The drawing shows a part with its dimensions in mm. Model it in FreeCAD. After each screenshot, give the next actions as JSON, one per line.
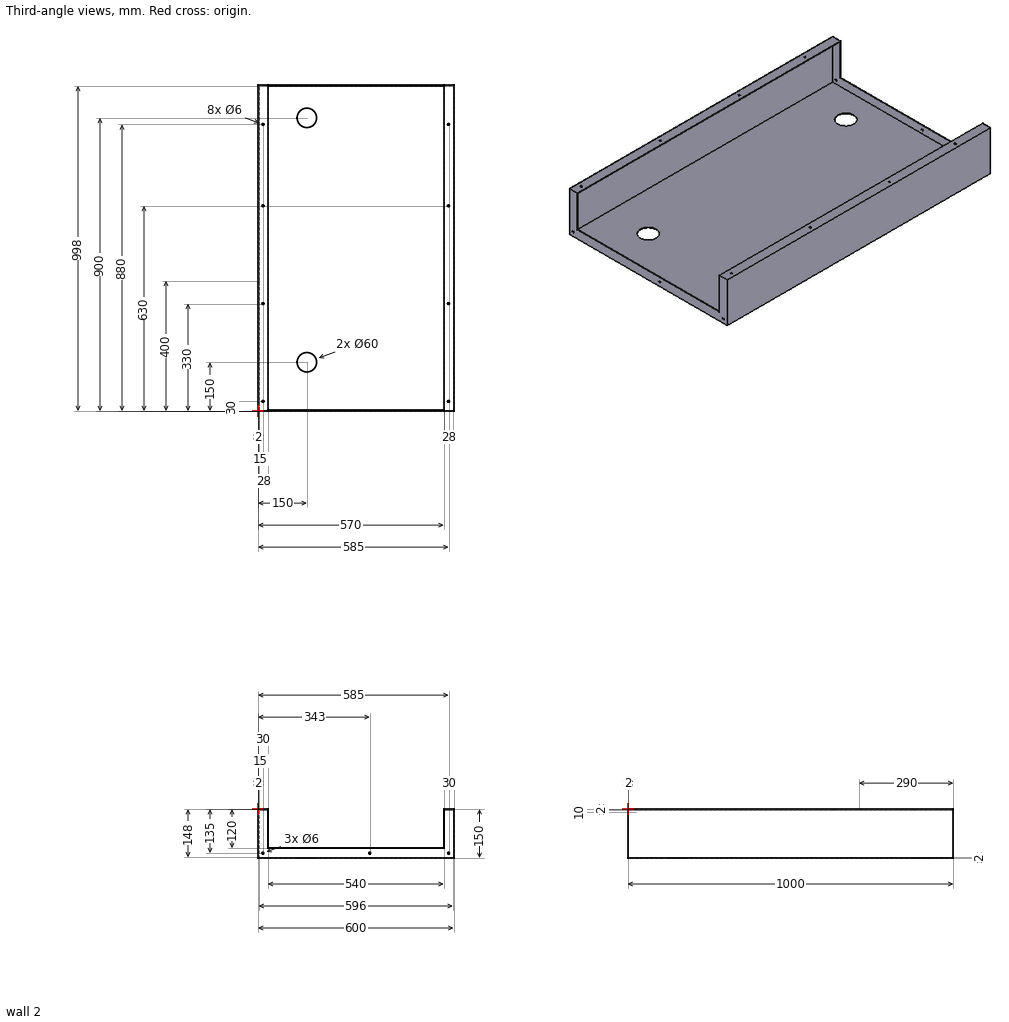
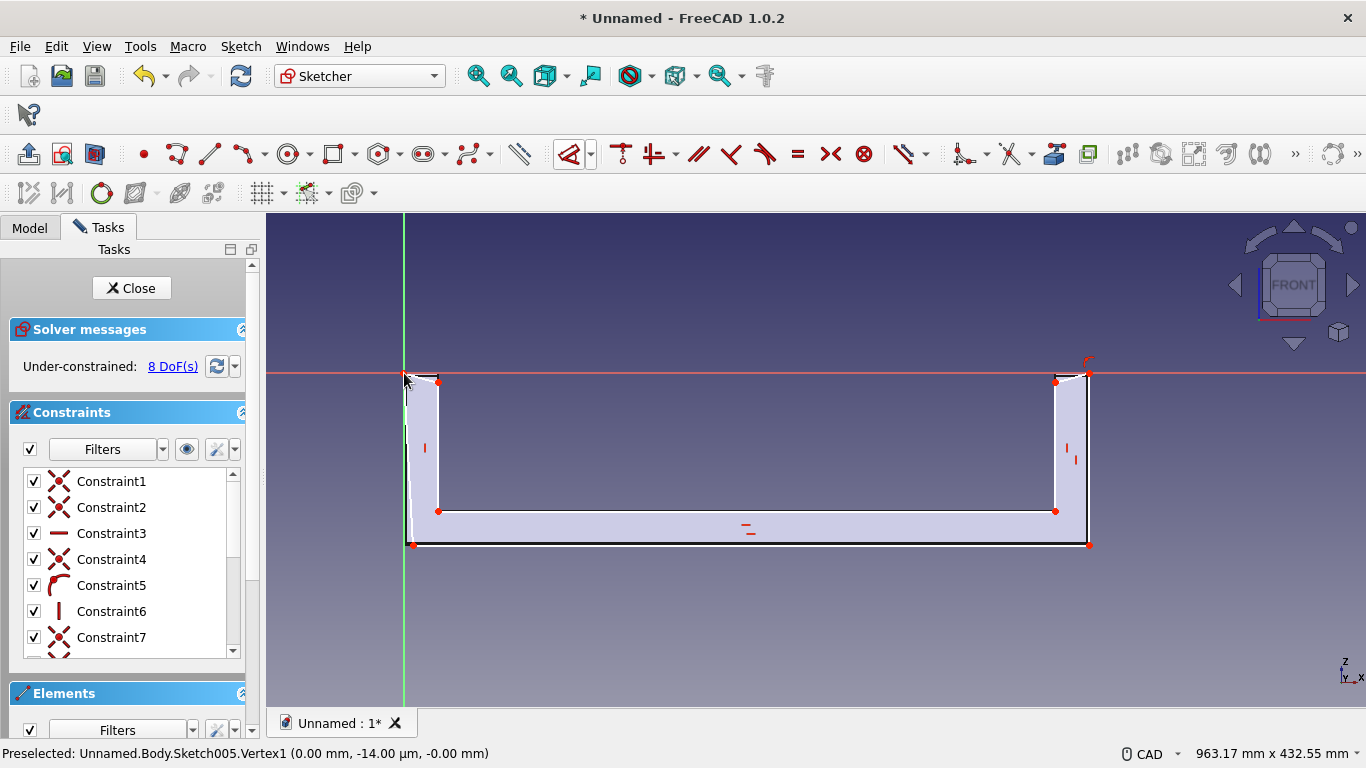
{"action": "left_click", "coordinate": [407, 425]}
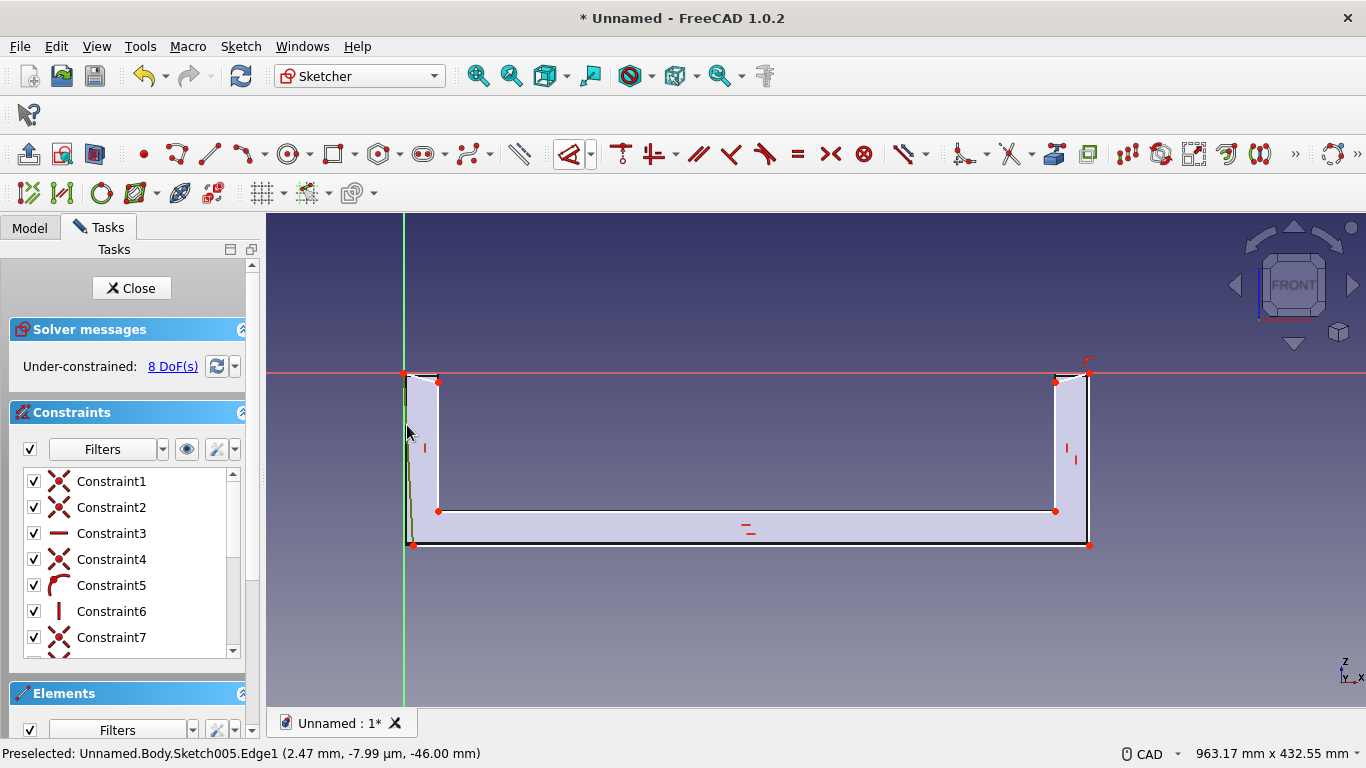
{"action": "left_click", "coordinate": [676, 154]}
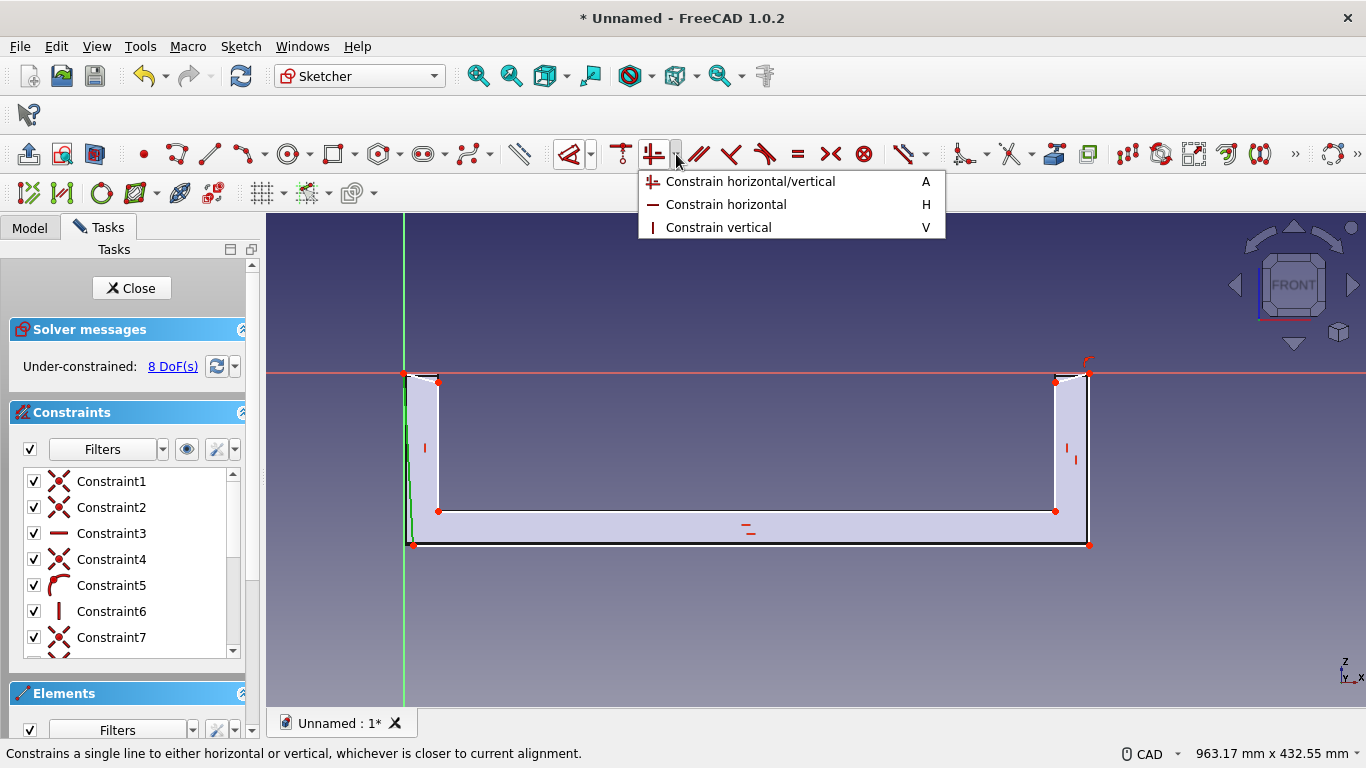
{"action": "left_click", "coordinate": [792, 228]}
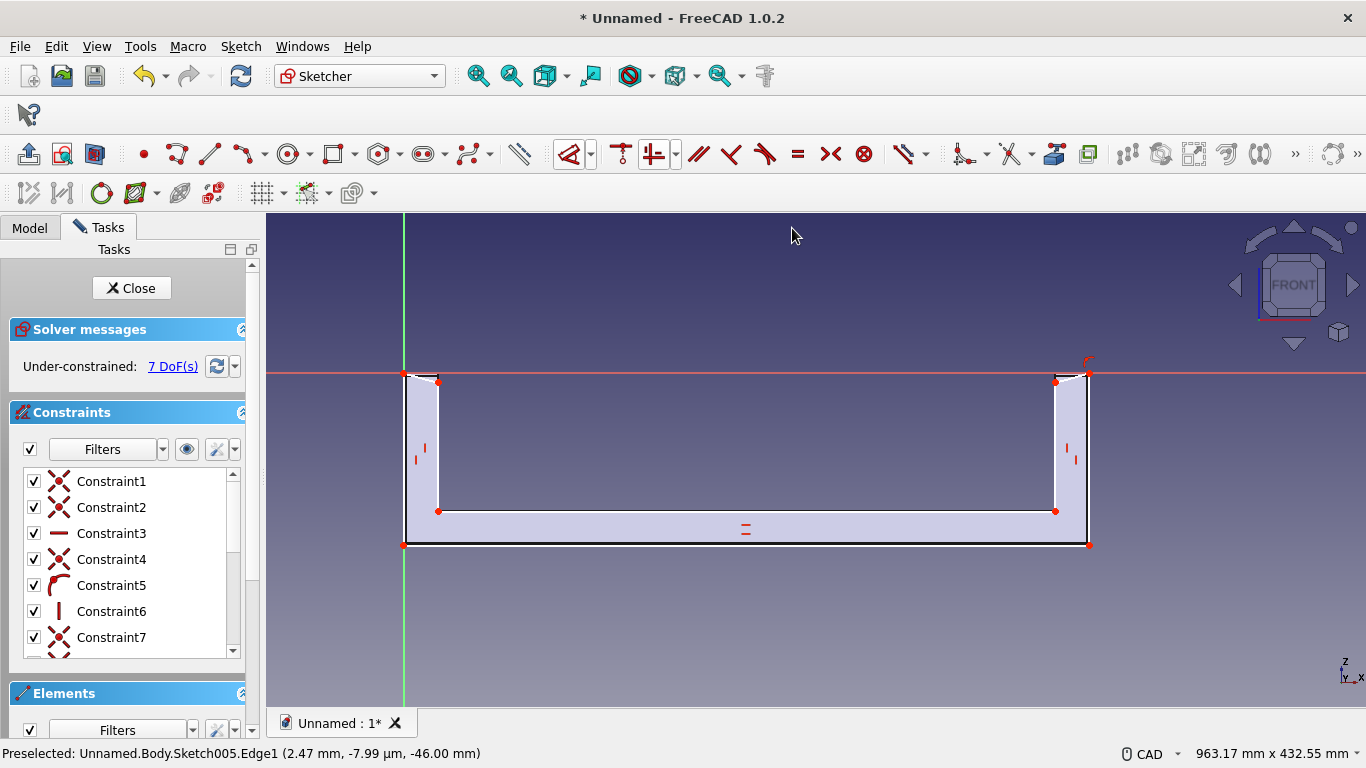
{"action": "scroll", "coordinate": [1079, 376], "scroll_direction": "up", "scroll_amount": 2}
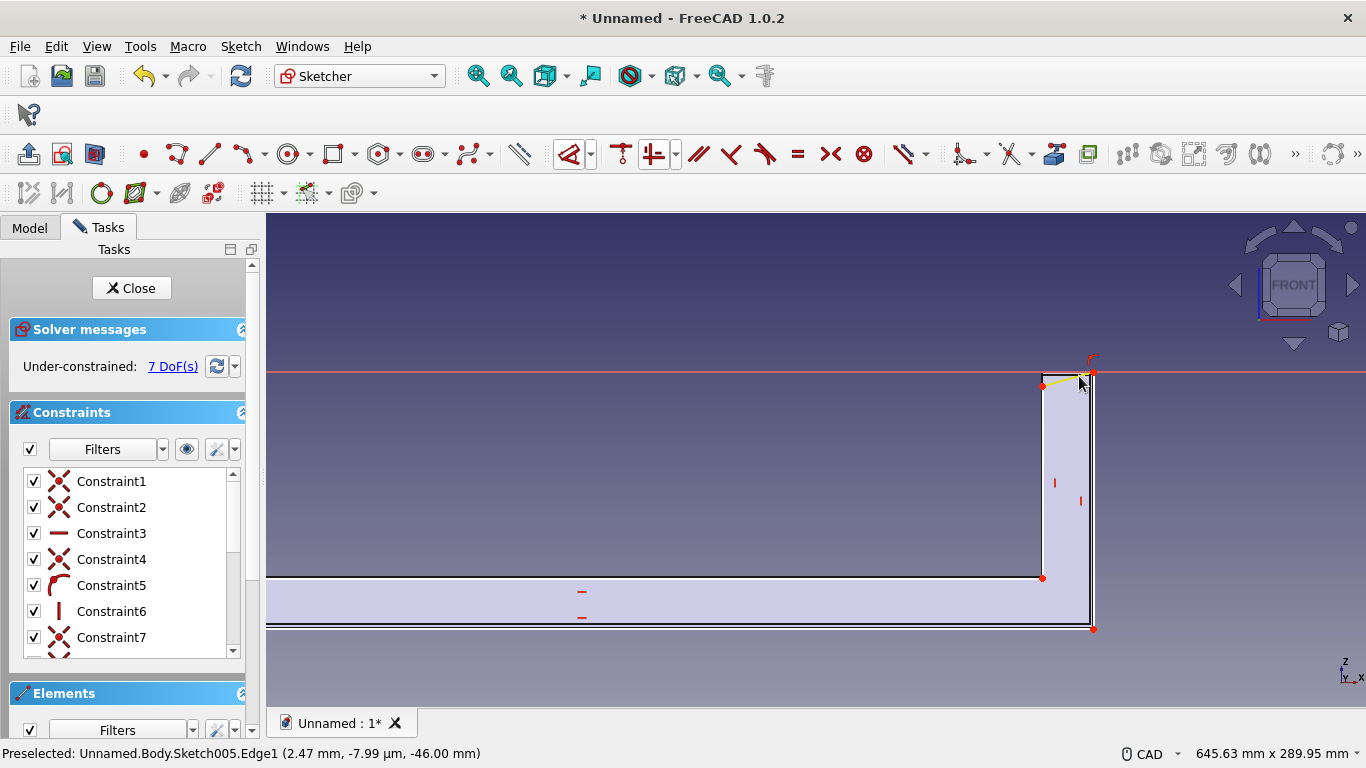
{"action": "left_click", "coordinate": [1078, 376]}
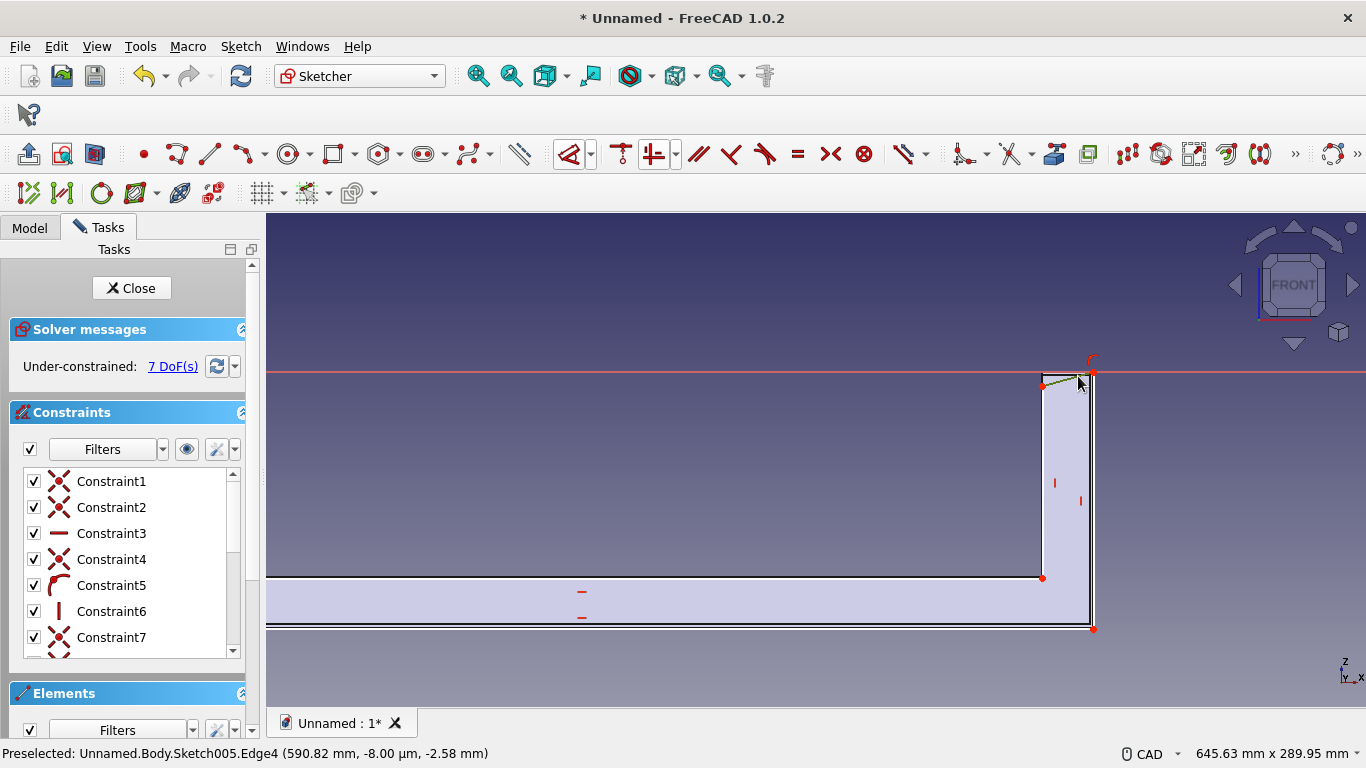
{"action": "key", "text": "h"}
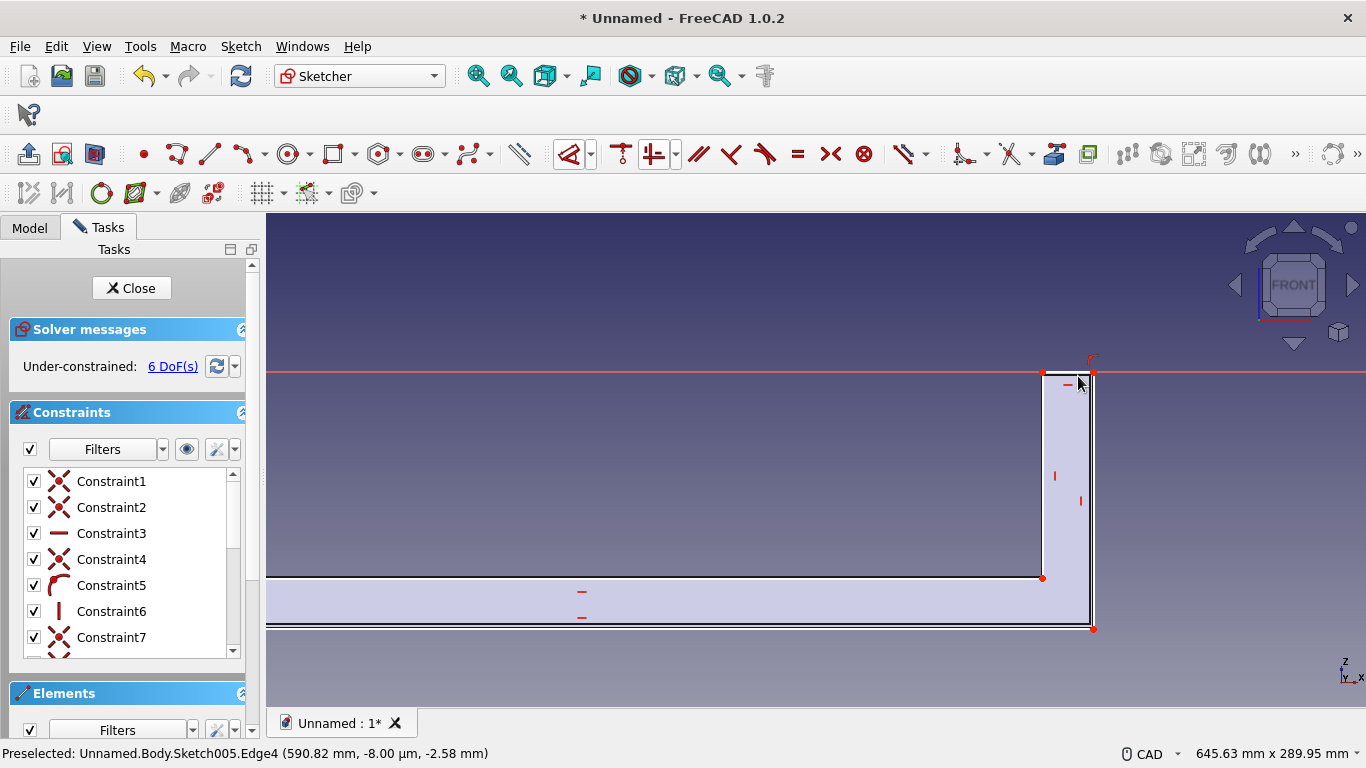
{"action": "scroll", "coordinate": [1083, 379], "scroll_direction": "down", "scroll_amount": 2}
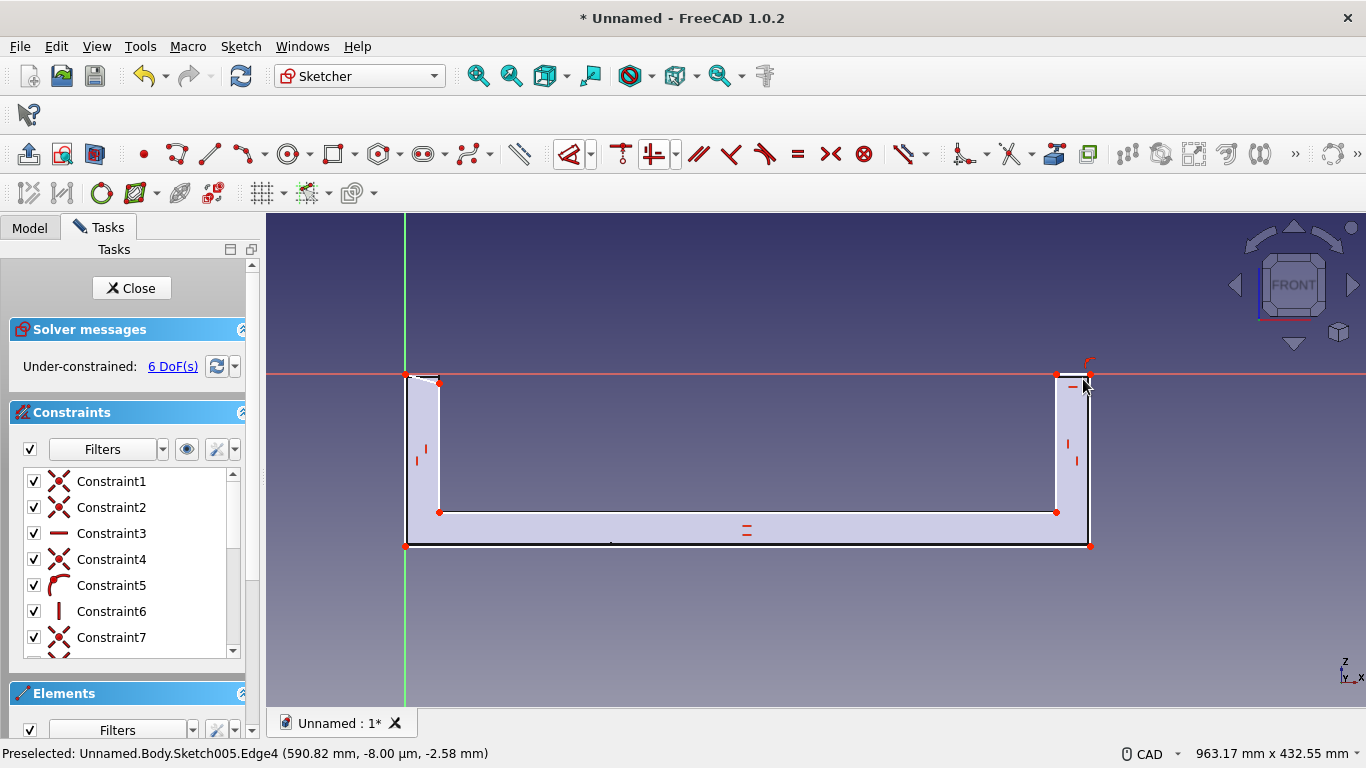
{"action": "scroll", "coordinate": [429, 381], "scroll_direction": "up", "scroll_amount": 4}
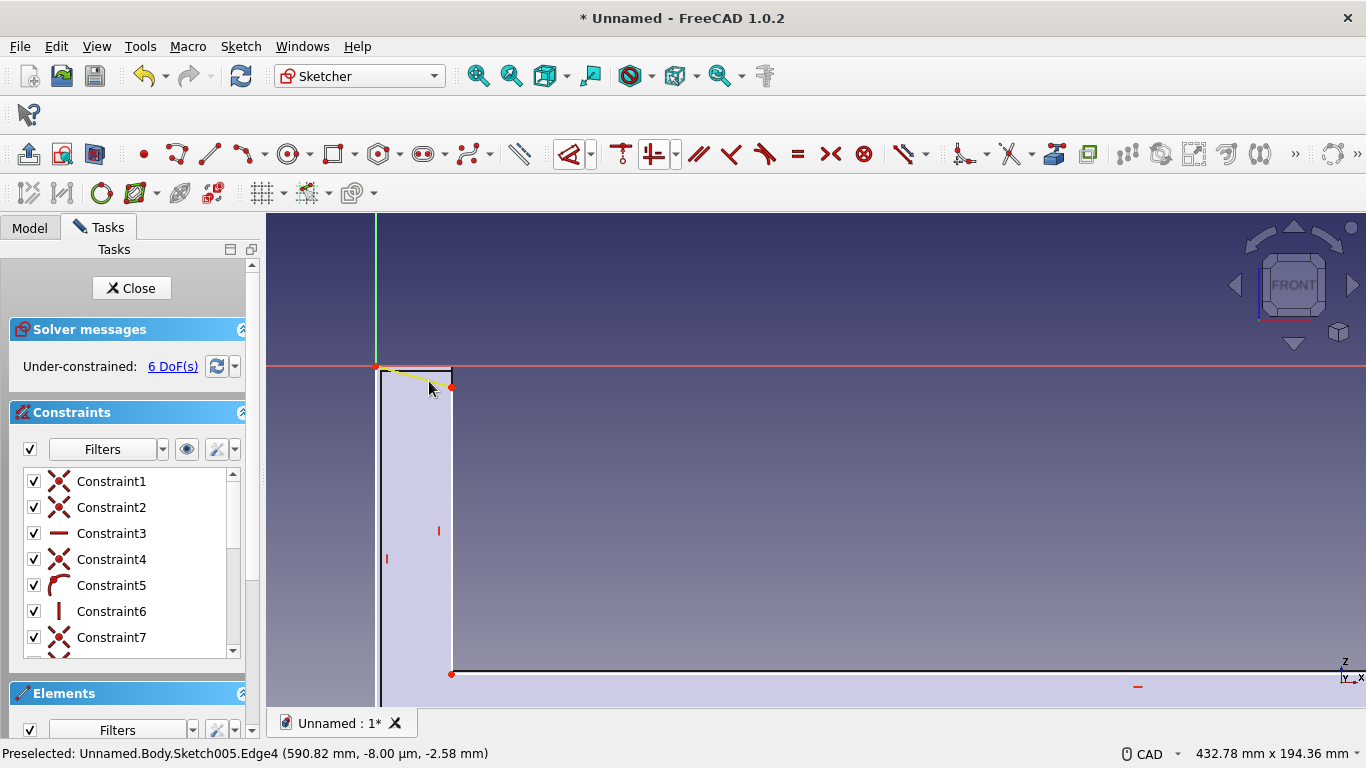
{"action": "left_click", "coordinate": [429, 381]}